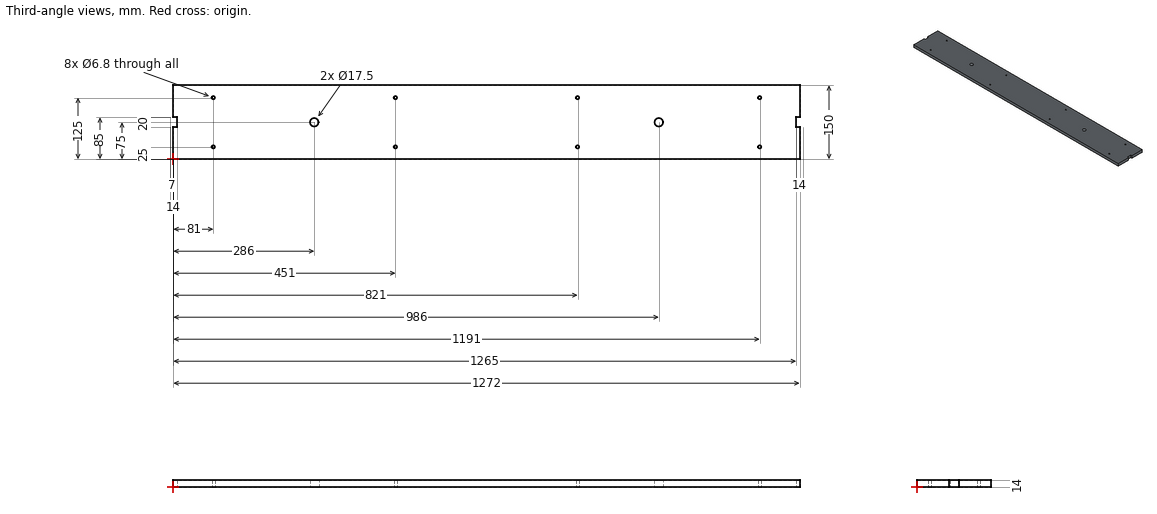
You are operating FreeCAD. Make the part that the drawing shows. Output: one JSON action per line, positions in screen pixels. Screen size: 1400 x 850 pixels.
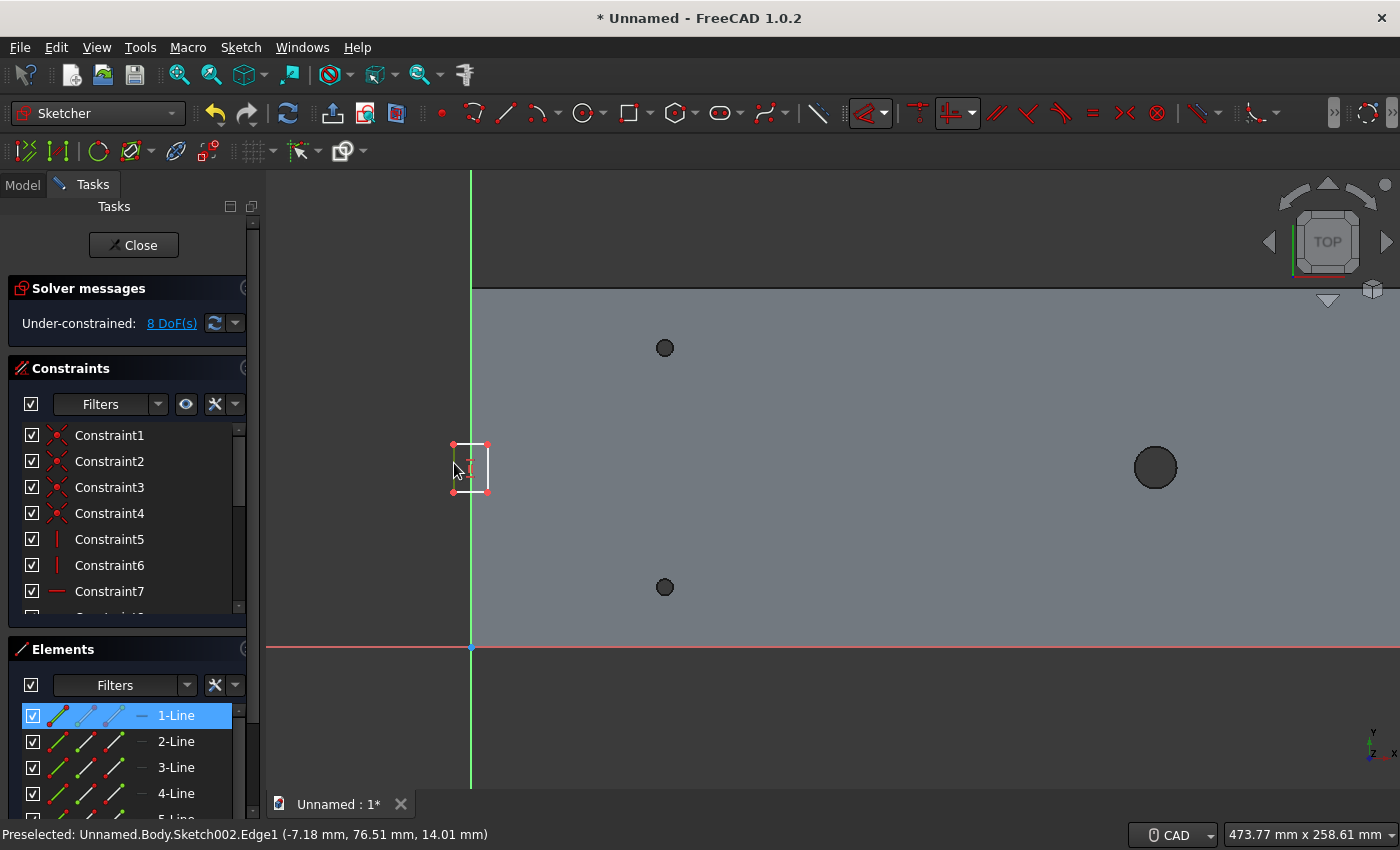
{"action": "left_click", "coordinate": [886, 114]}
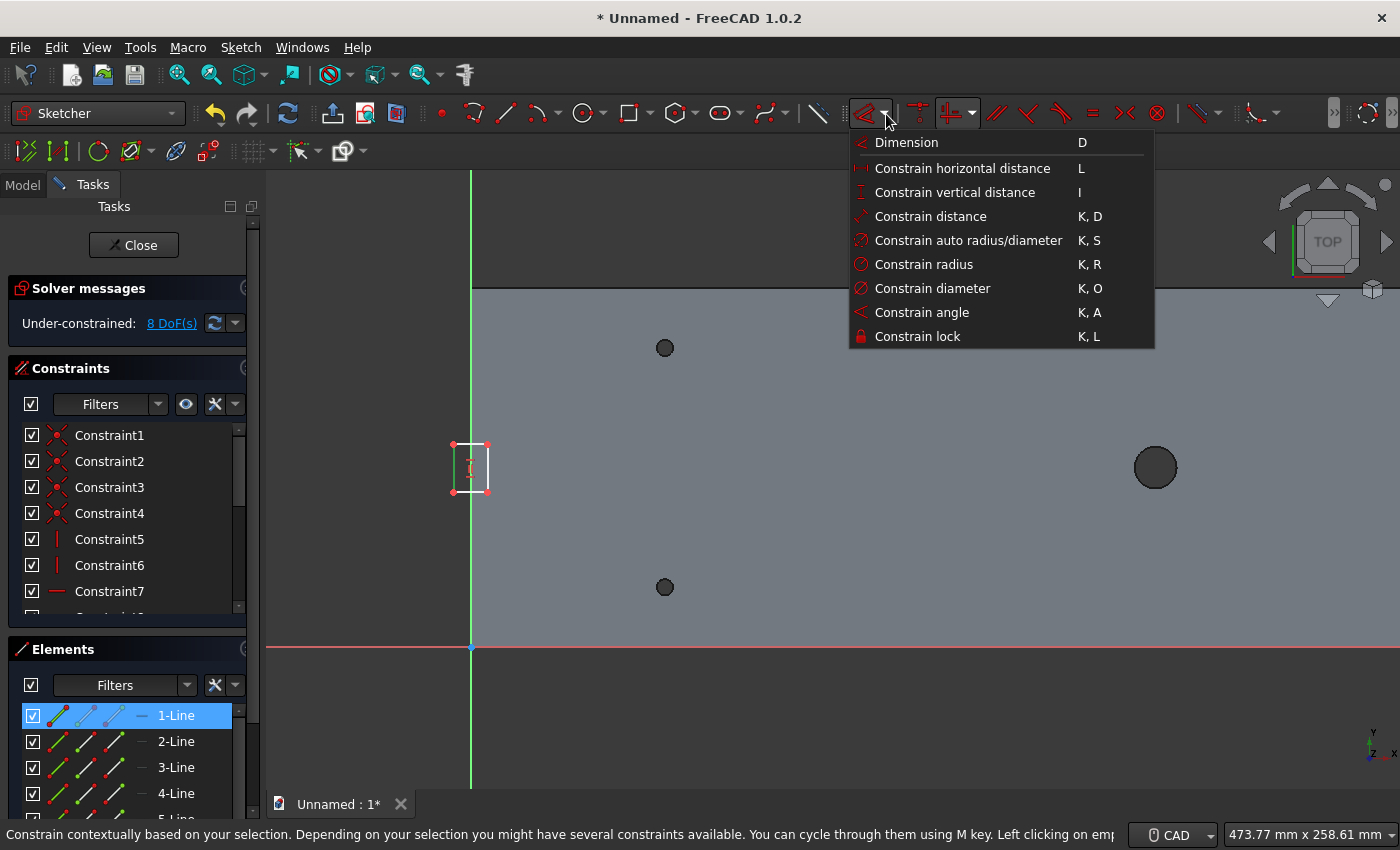
{"action": "left_click", "coordinate": [1002, 192]}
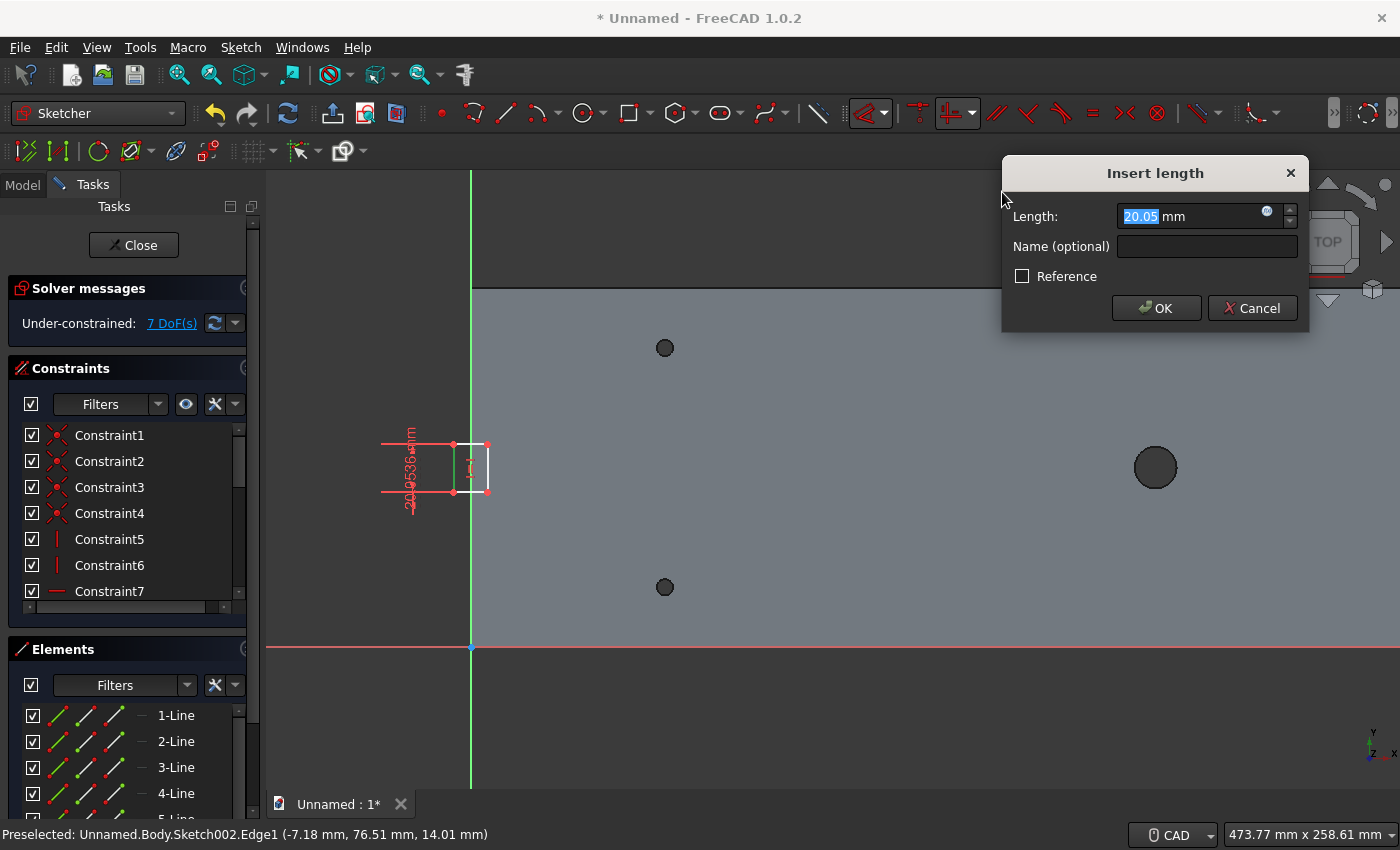
{"action": "type", "text": "20"}
{"action": "key", "text": "Return"}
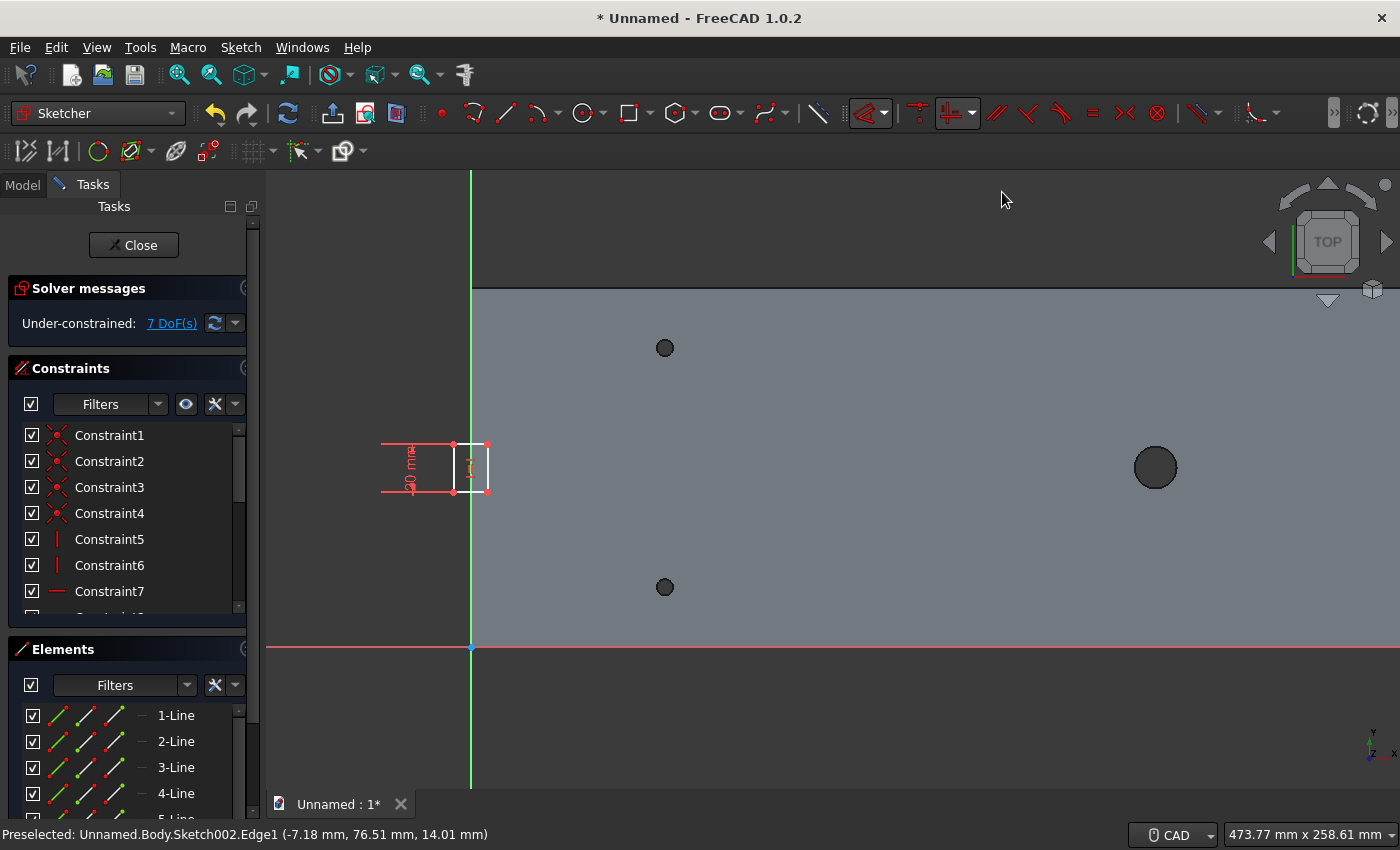
{"action": "left_click", "coordinate": [468, 492]}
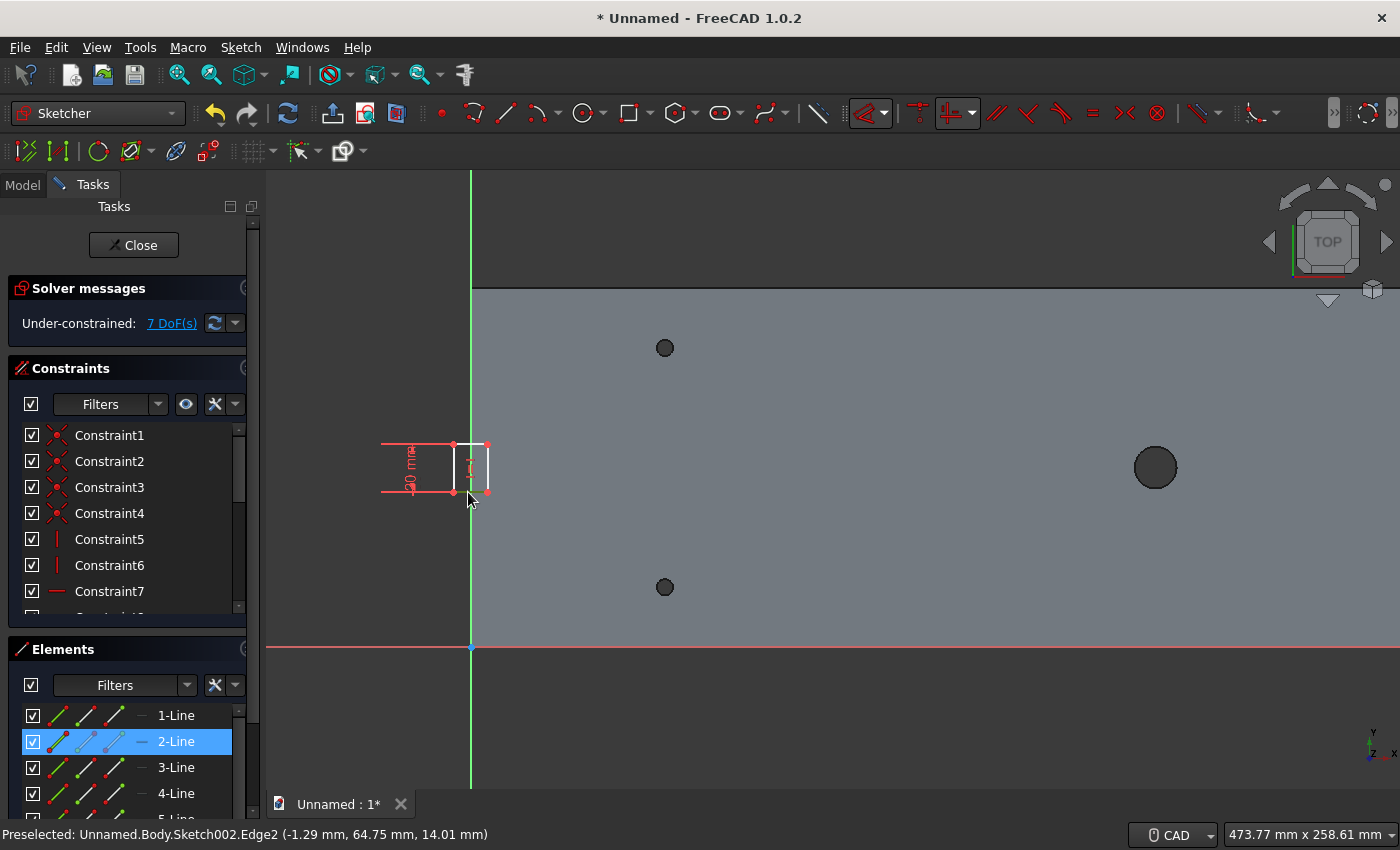
{"action": "left_click", "coordinate": [886, 114]}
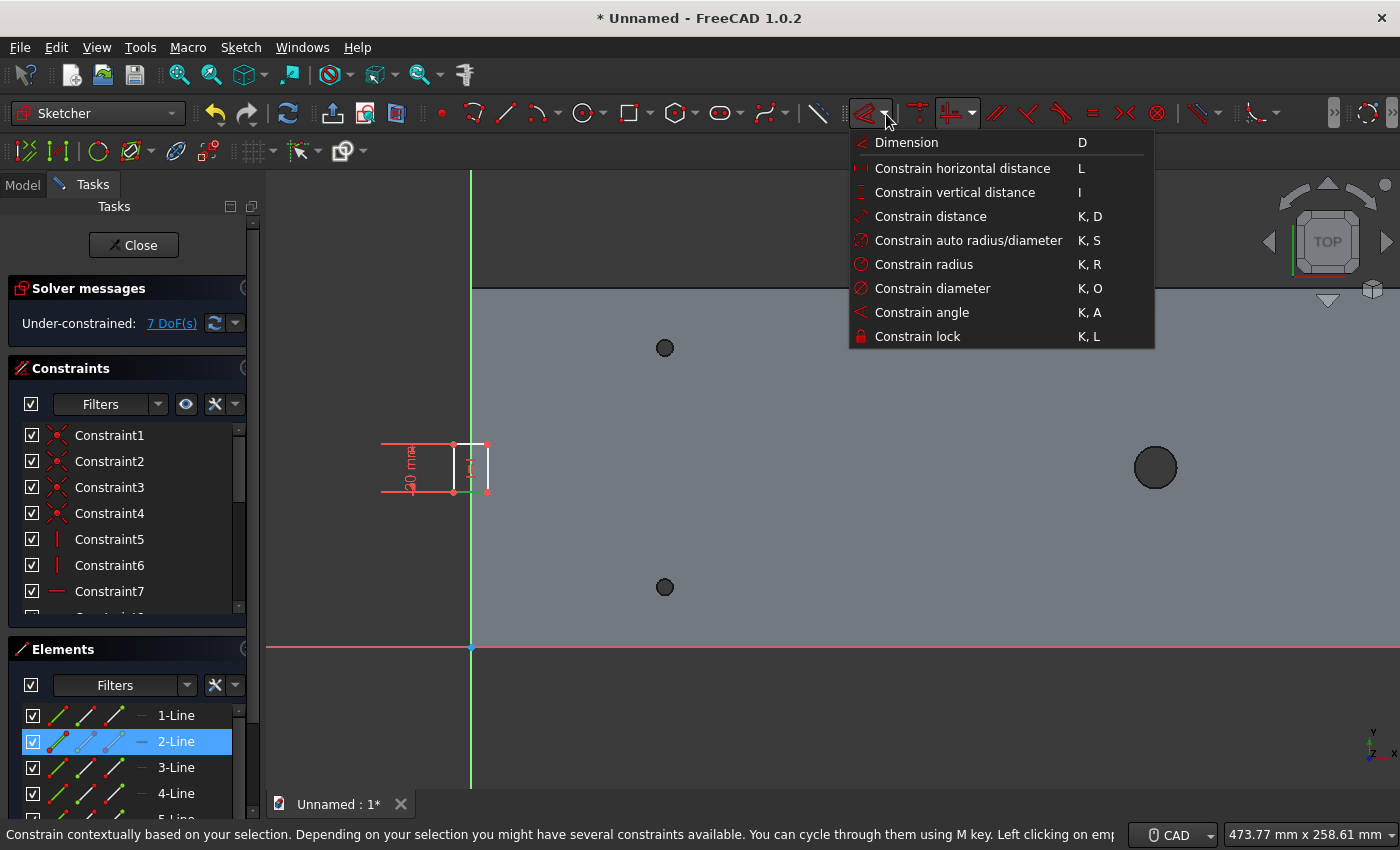
{"action": "left_click", "coordinate": [1002, 168]}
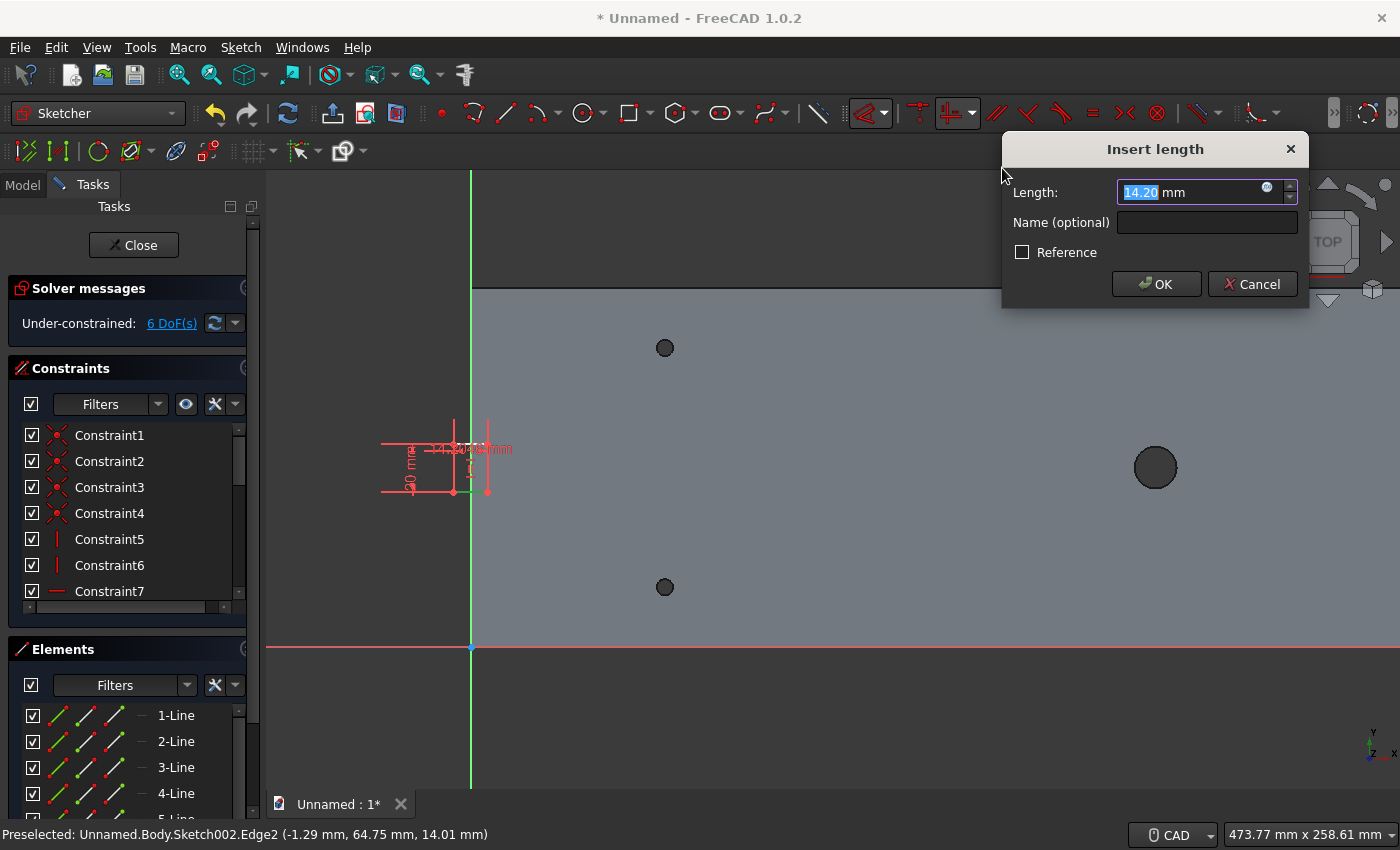
{"action": "type", "text": "14"}
{"action": "key", "text": "Return"}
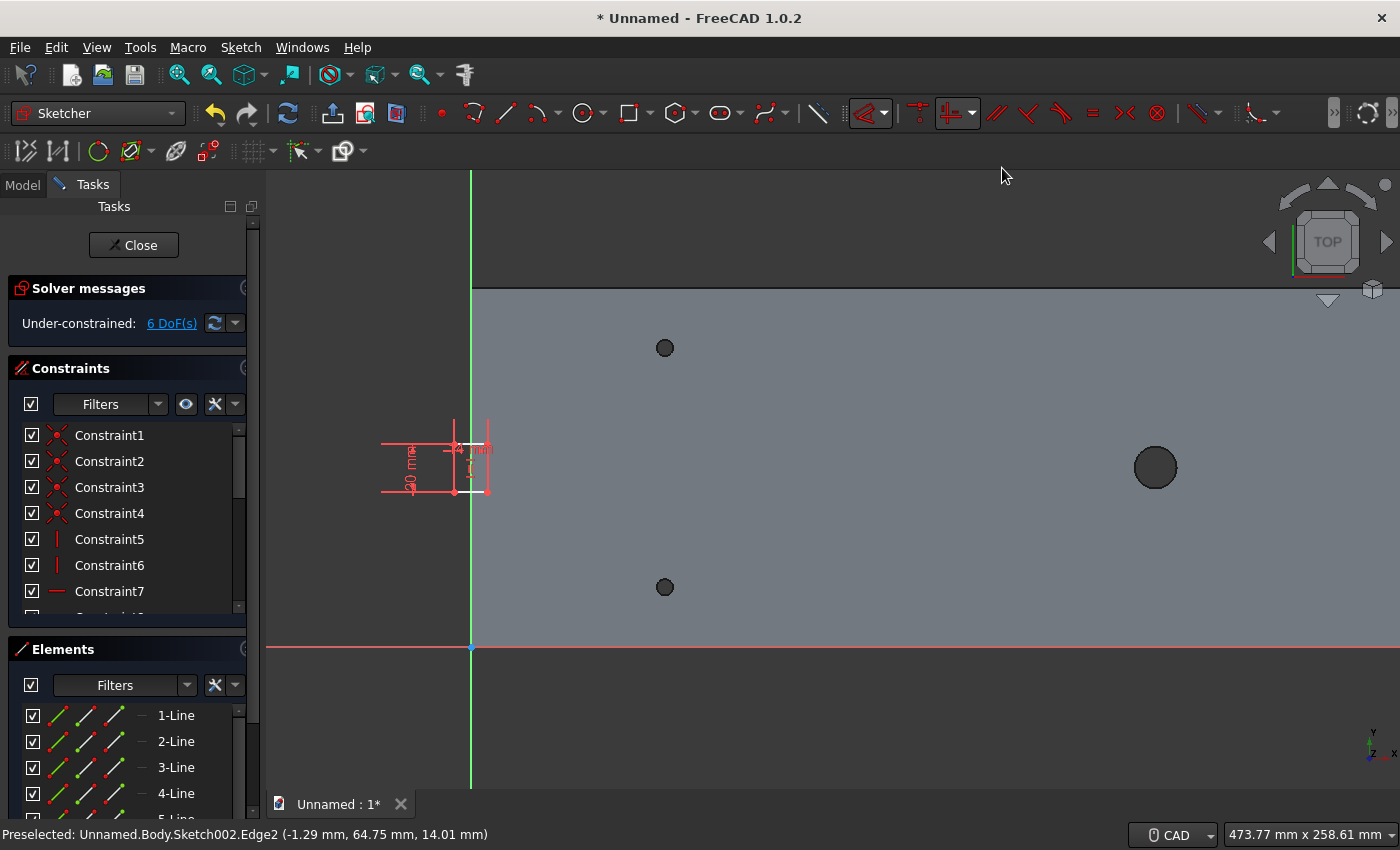
{"action": "scroll", "coordinate": [454, 463], "scroll_direction": "down", "scroll_amount": 8}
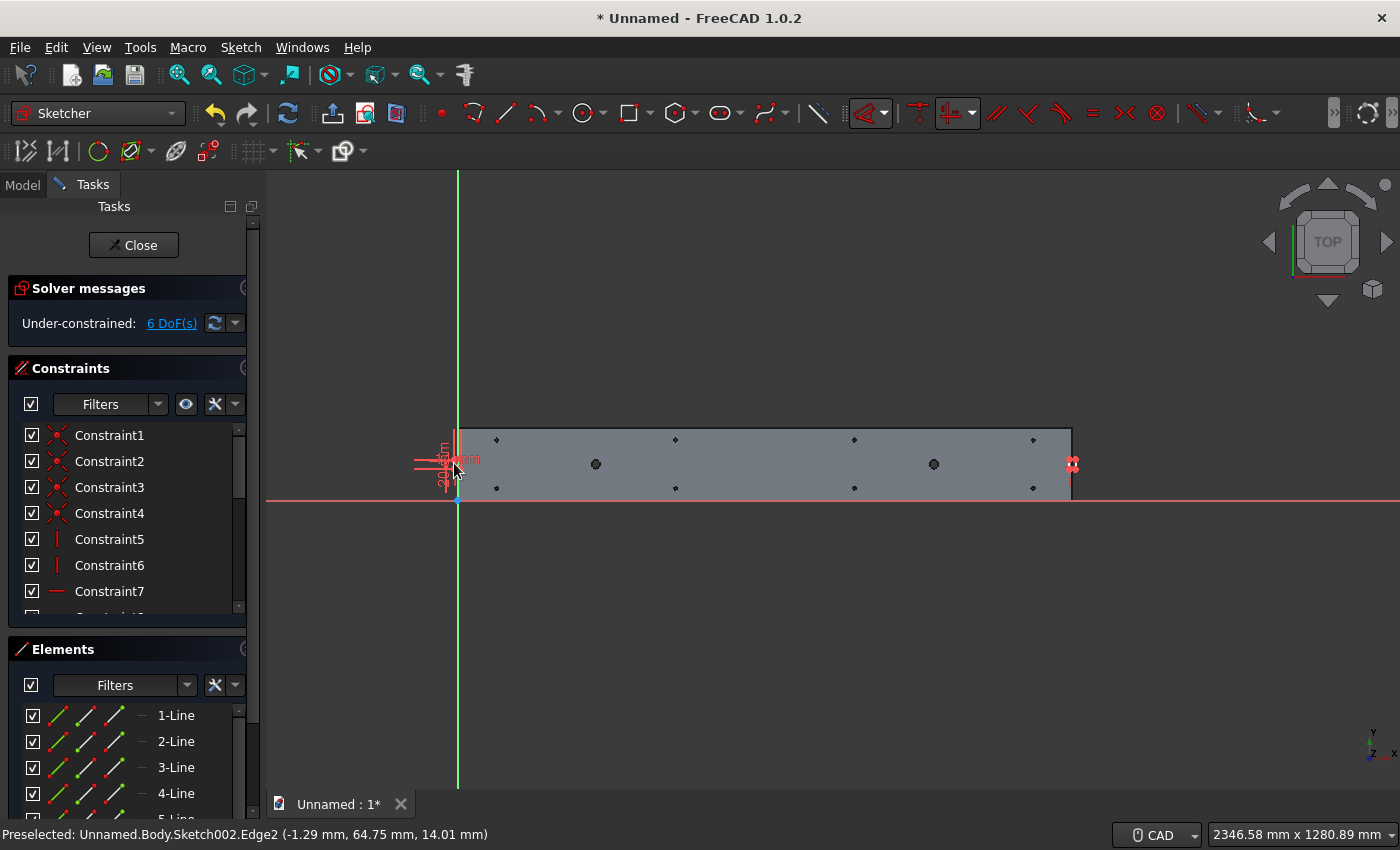
{"action": "scroll", "coordinate": [1069, 463], "scroll_direction": "up", "scroll_amount": 8}